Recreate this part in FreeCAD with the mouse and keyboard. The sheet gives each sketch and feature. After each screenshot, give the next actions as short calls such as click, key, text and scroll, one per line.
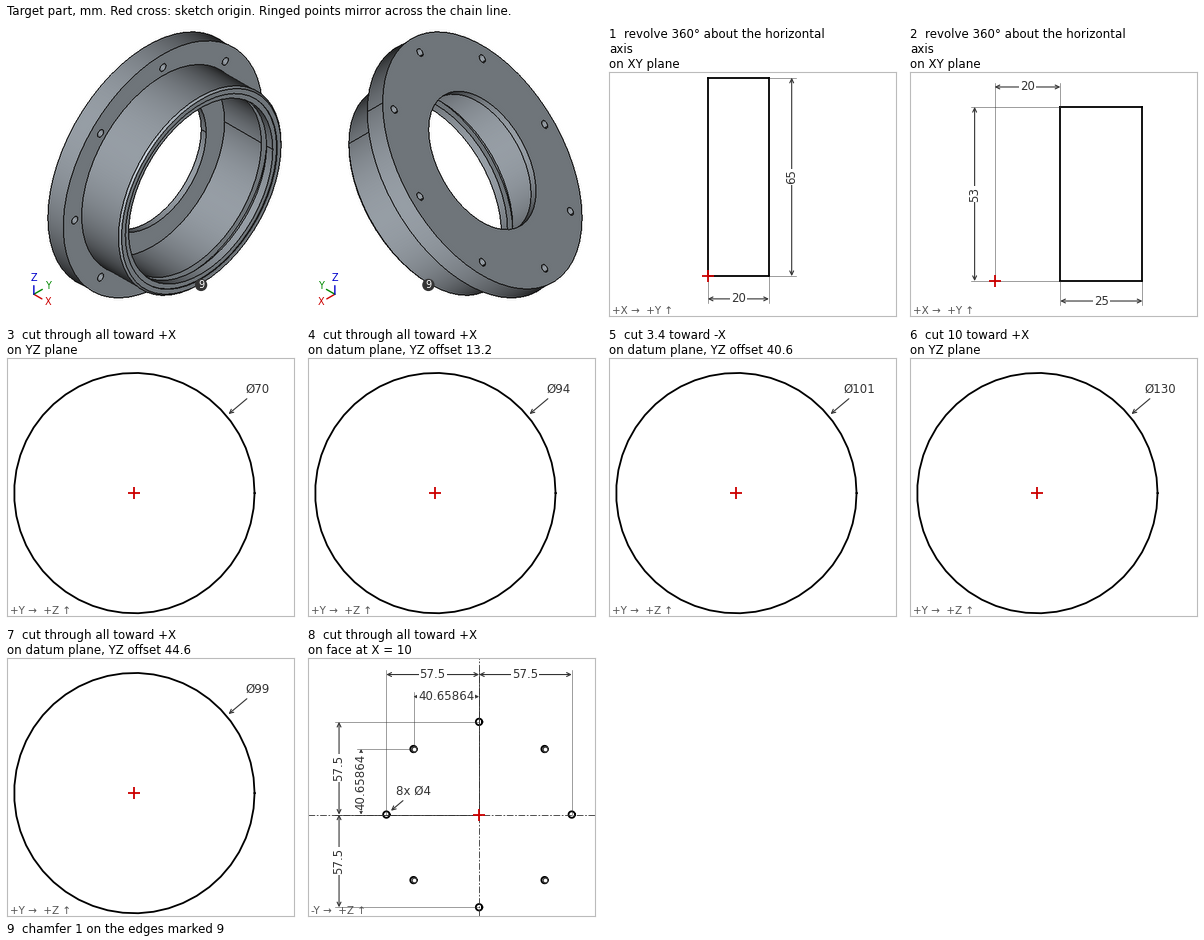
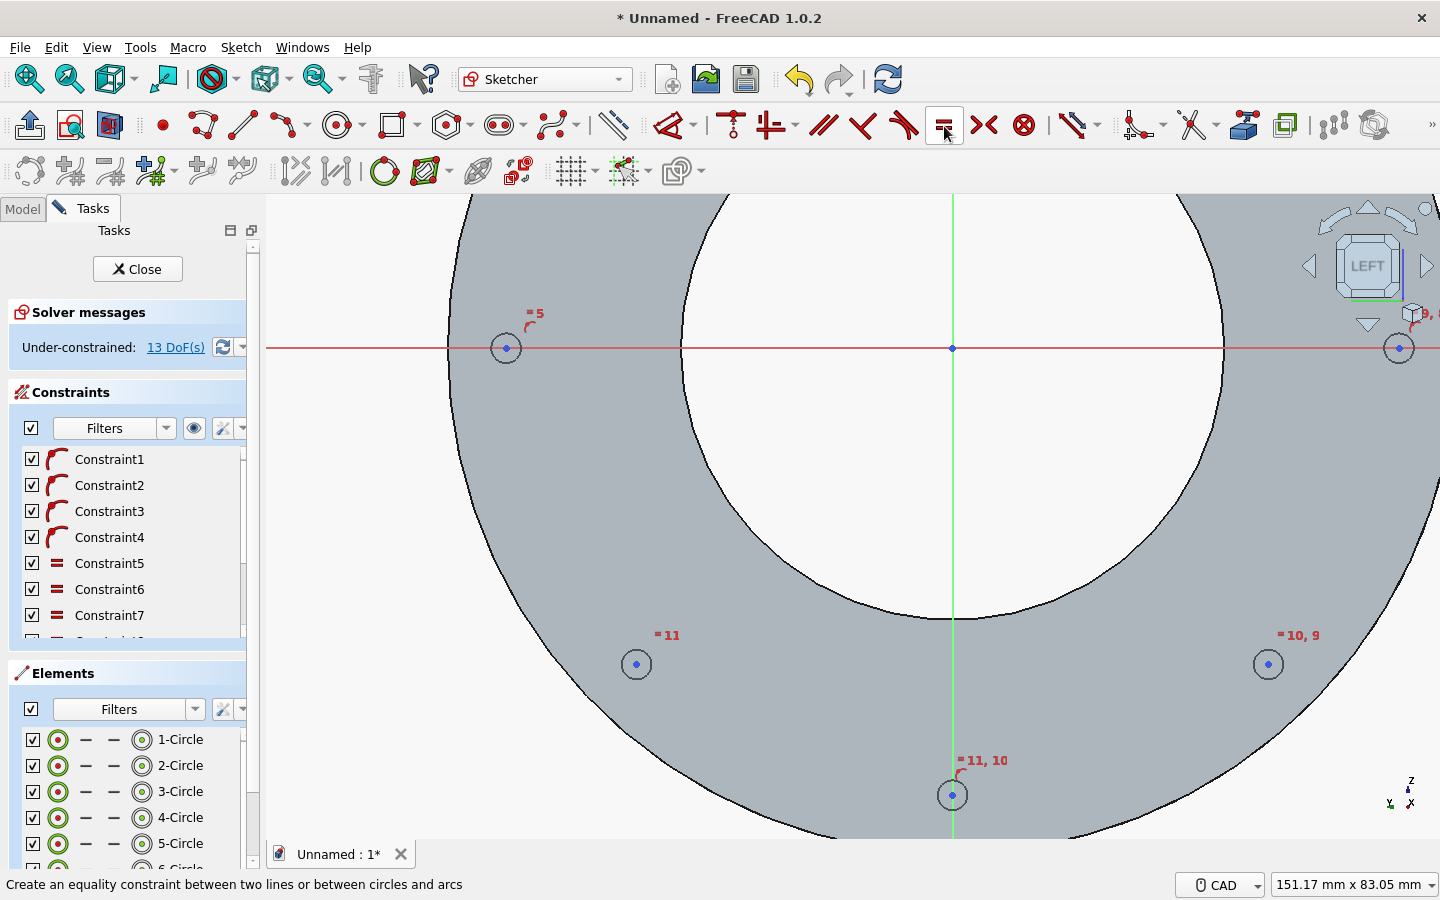
scroll(647, 654, down, 4)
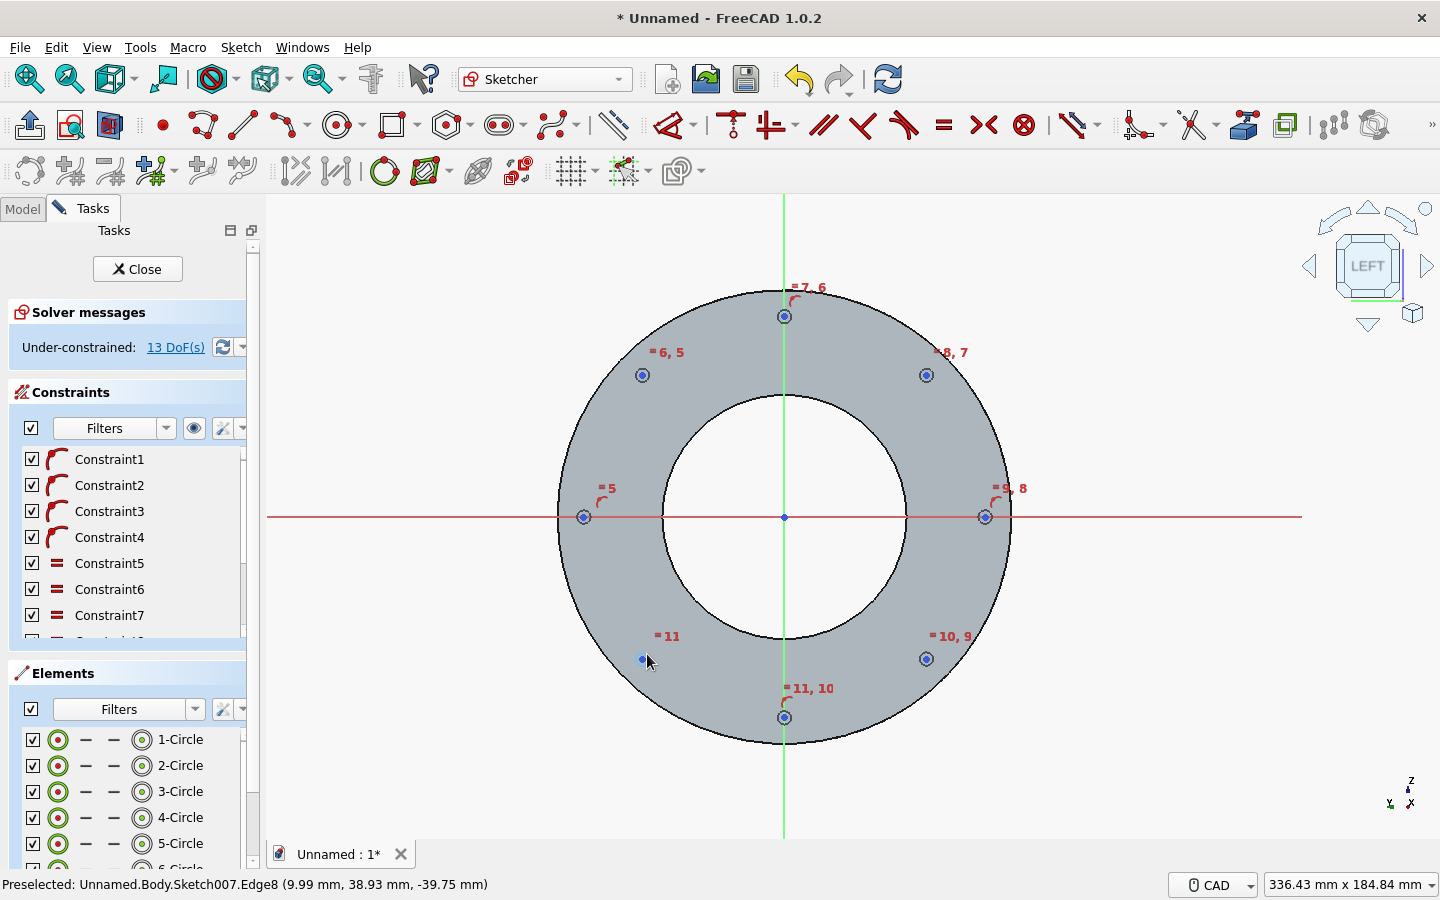
click(643, 375)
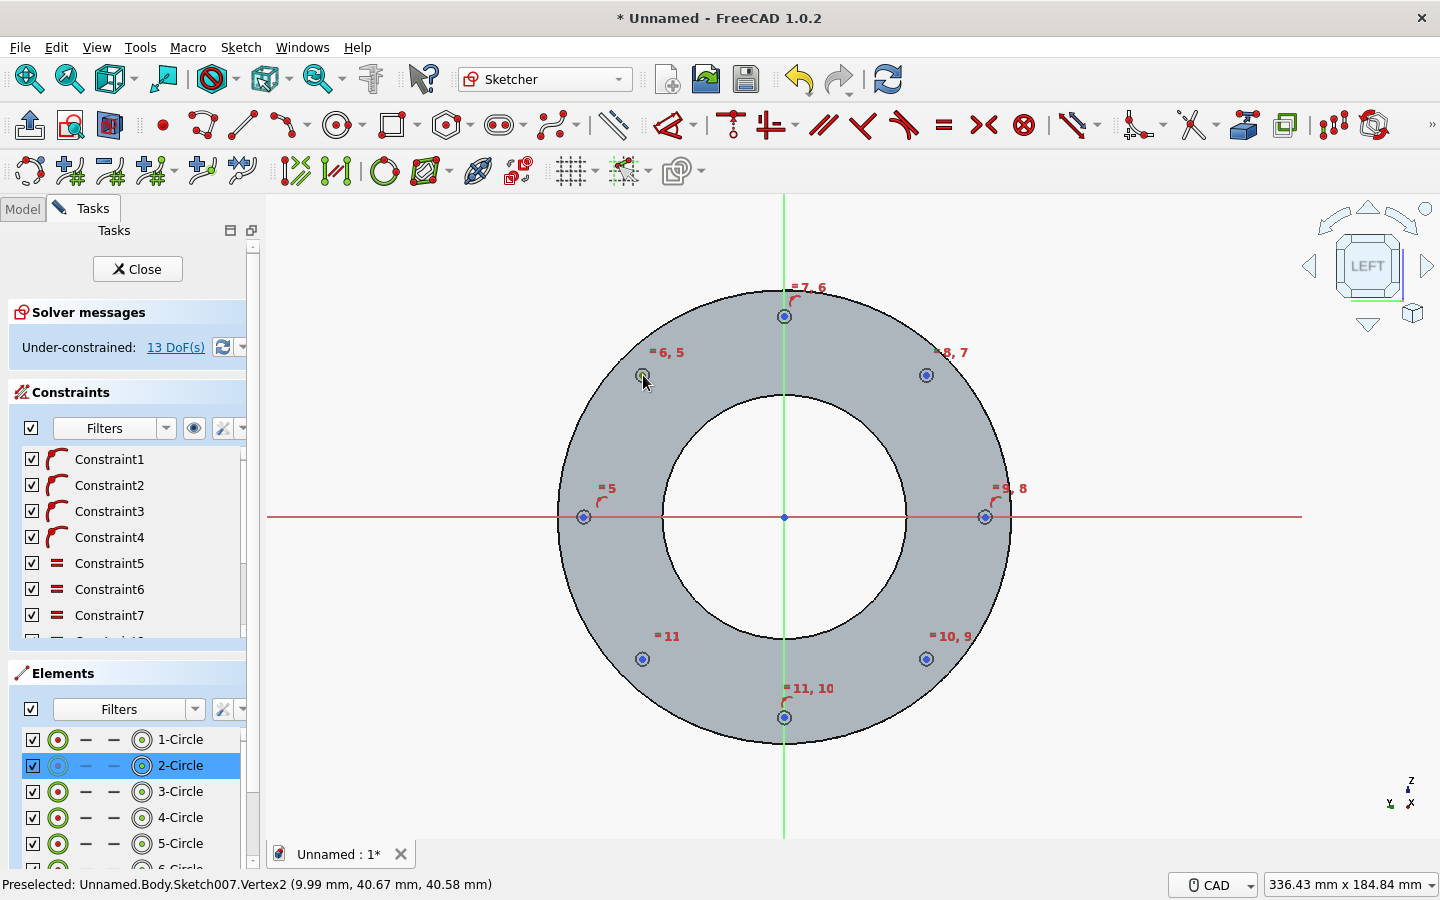
click(927, 375)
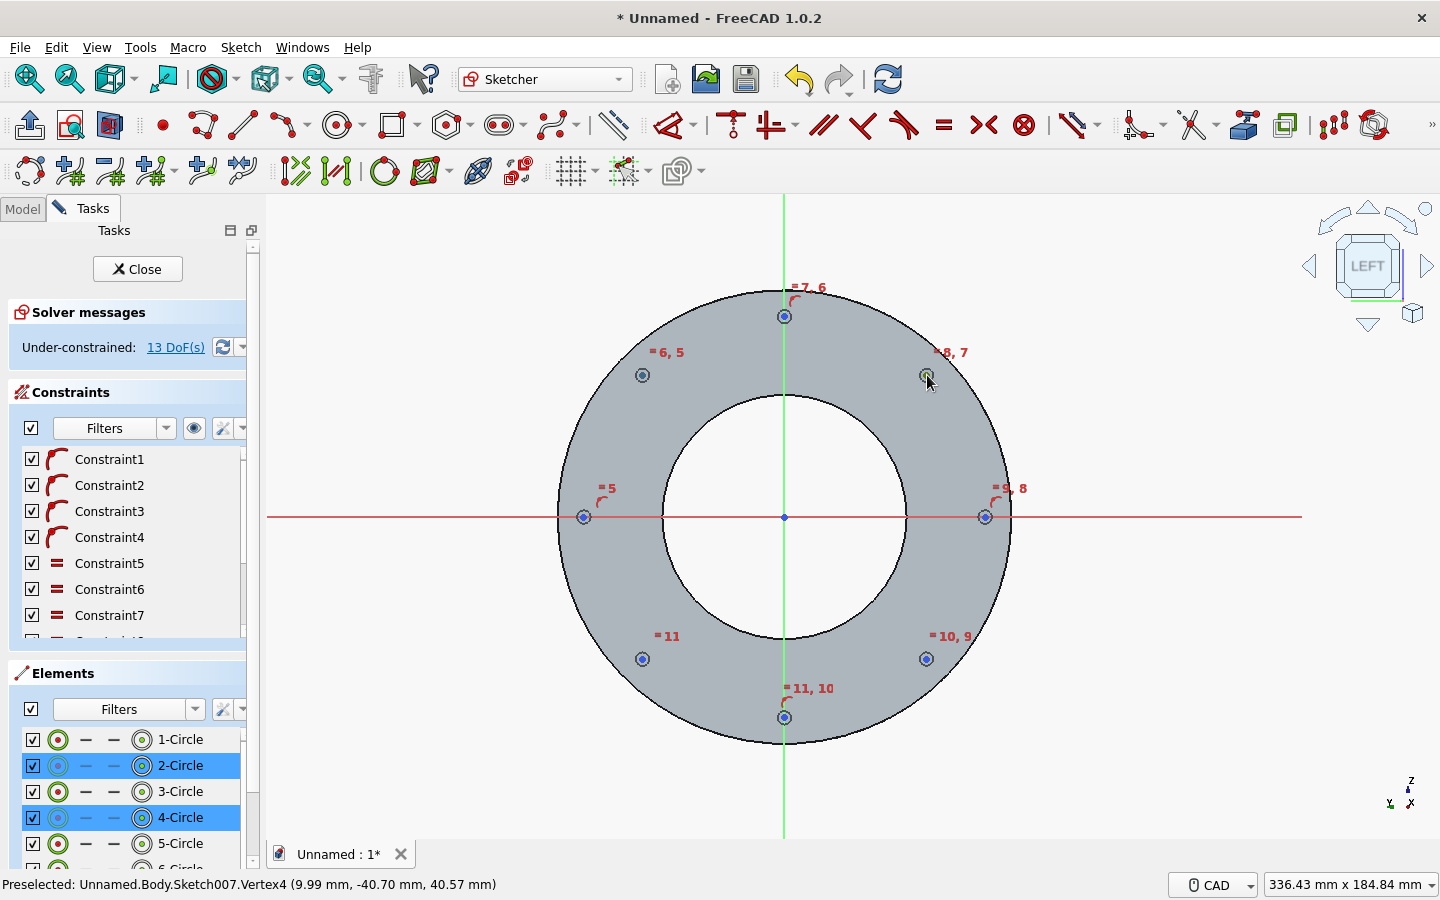
click(784, 769)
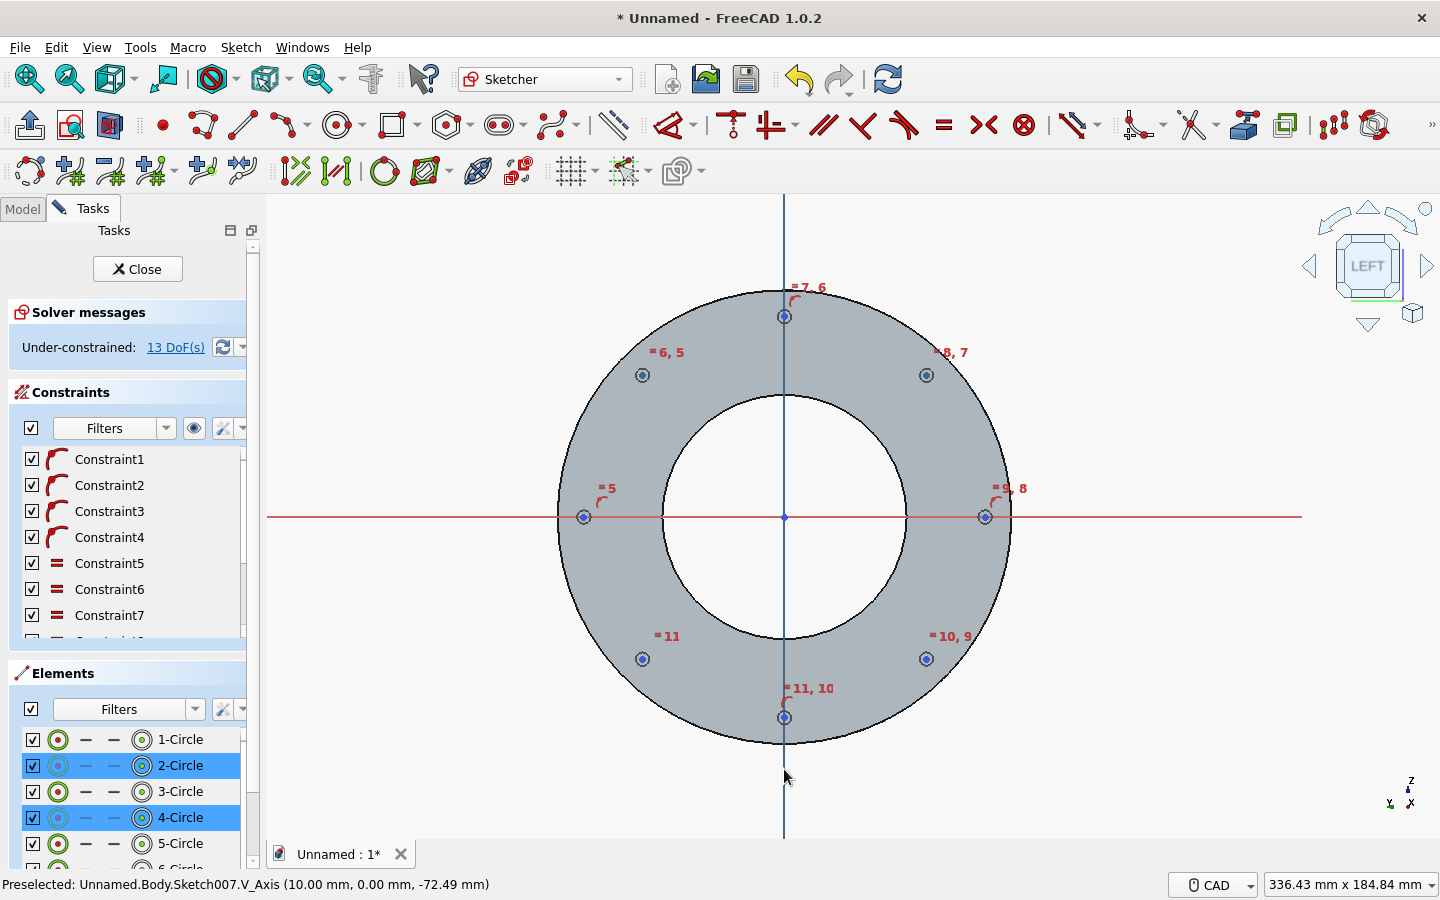
click(984, 126)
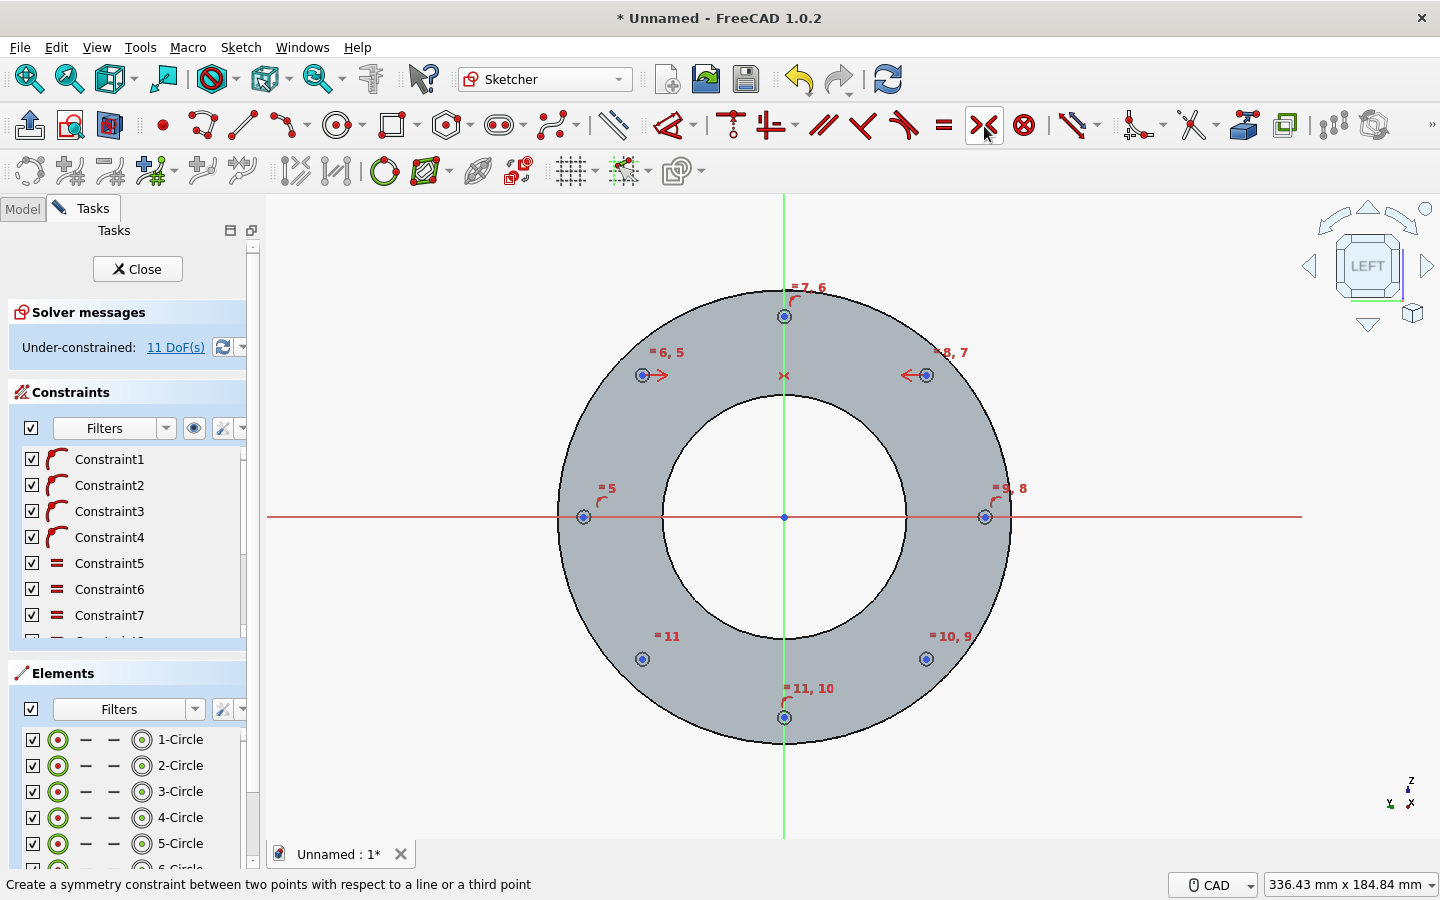
click(927, 375)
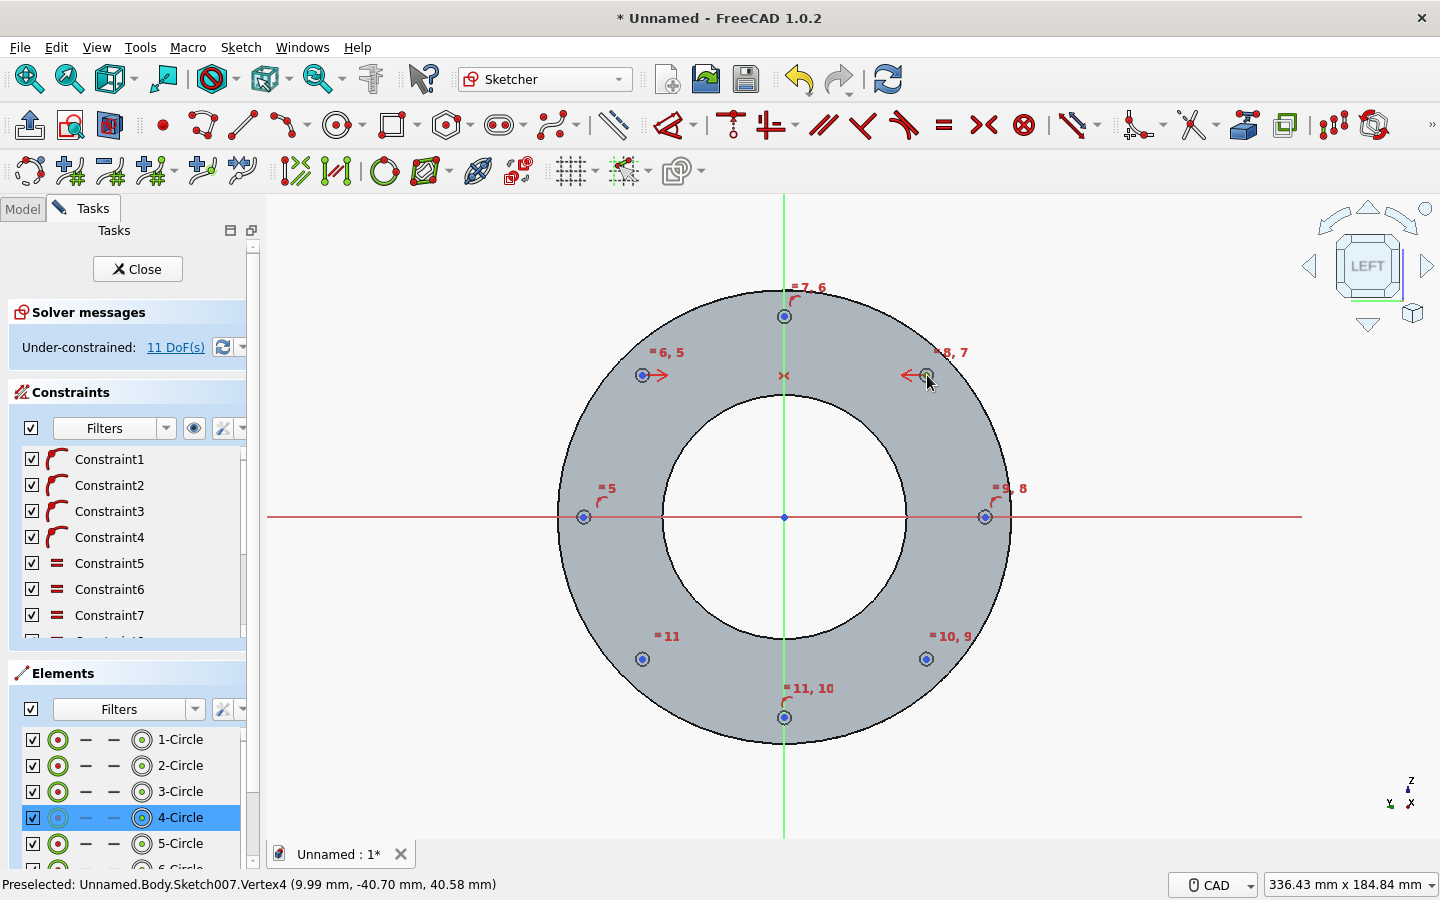
click(926, 659)